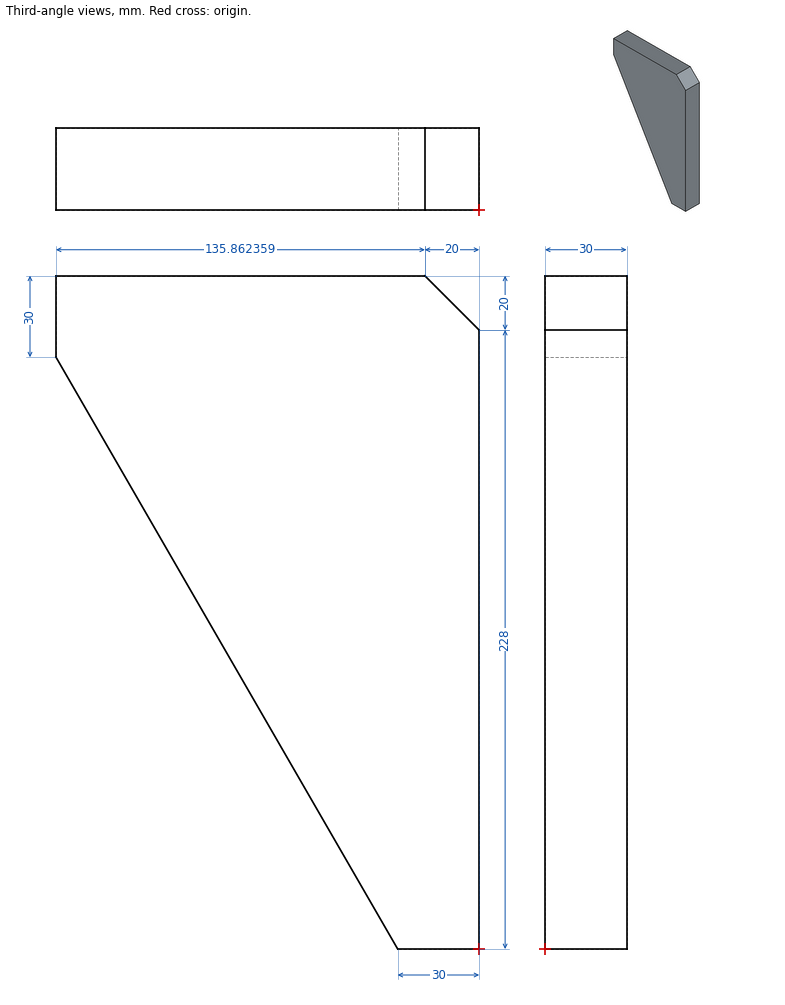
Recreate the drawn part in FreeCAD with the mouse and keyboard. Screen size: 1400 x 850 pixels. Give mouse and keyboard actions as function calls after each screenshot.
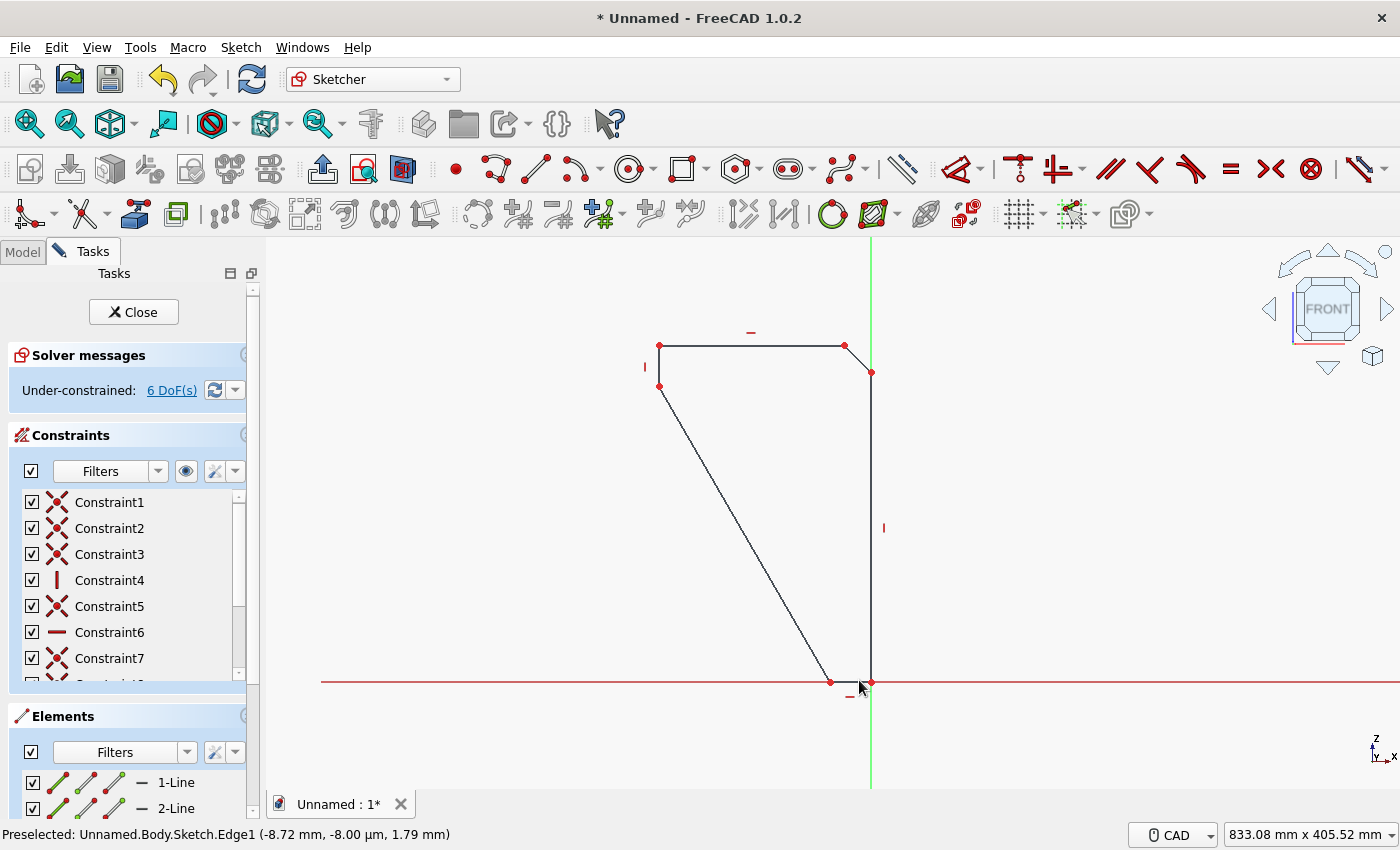
click(956, 170)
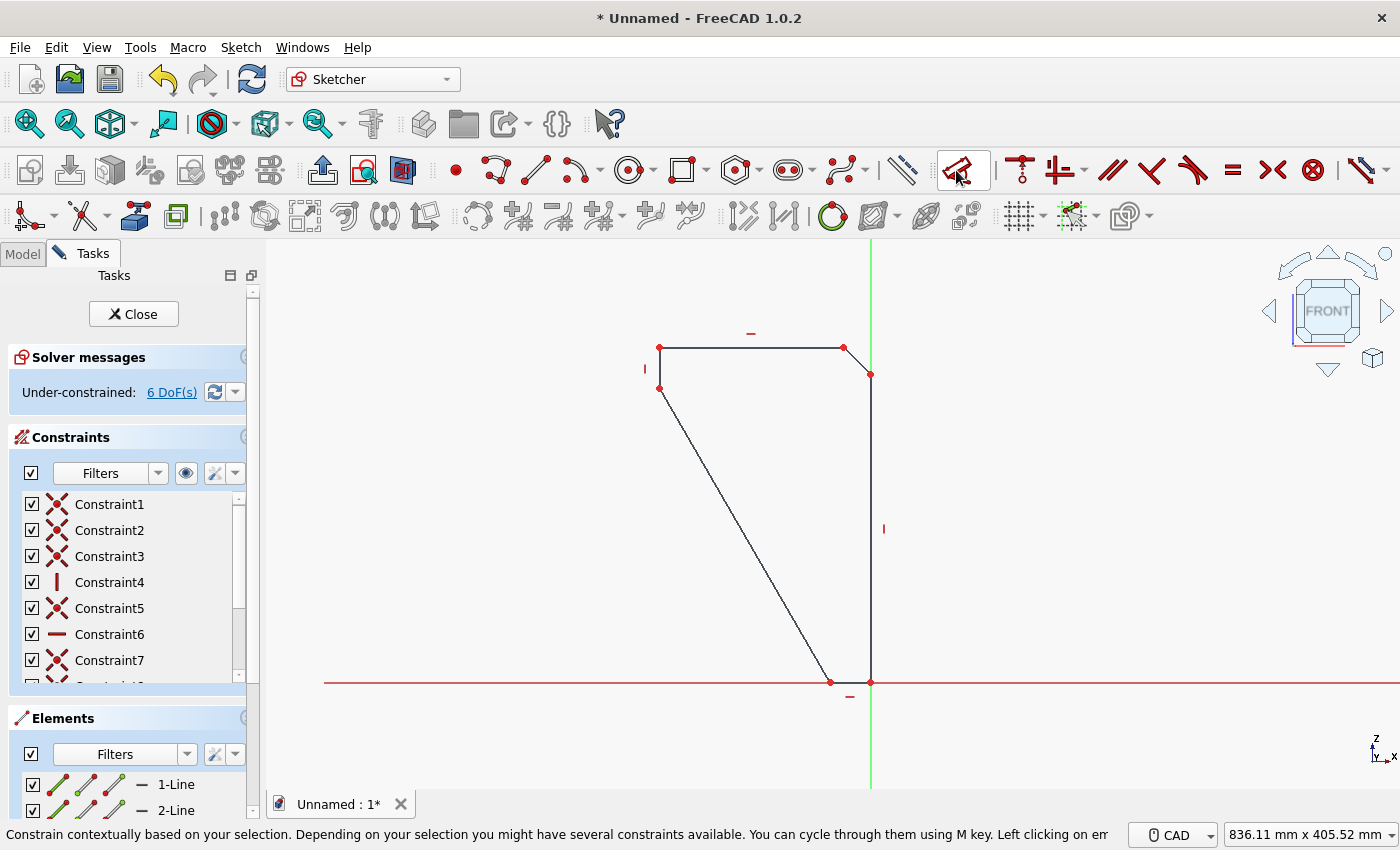
click(859, 683)
click(850, 717)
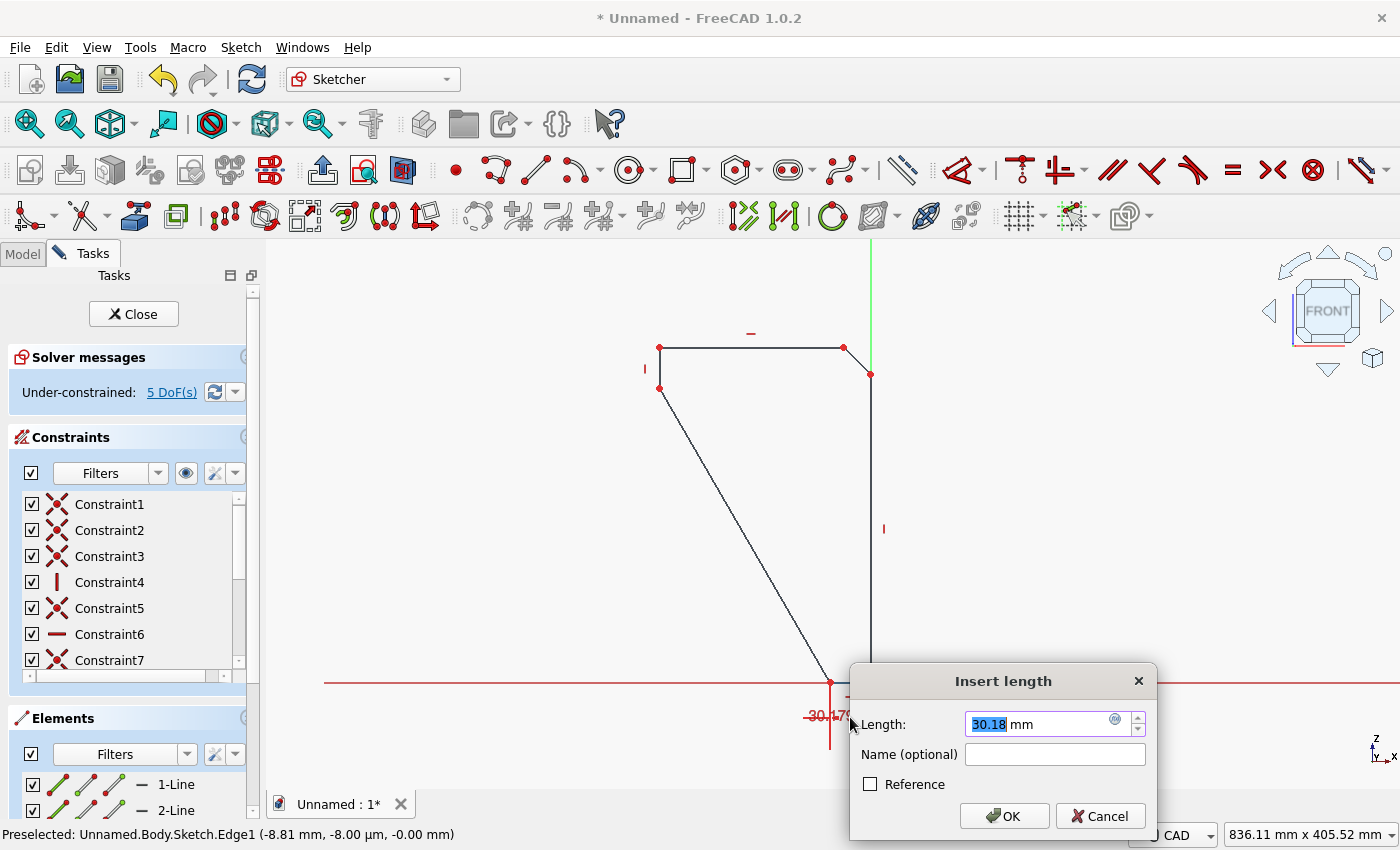
text(30)
key(Return)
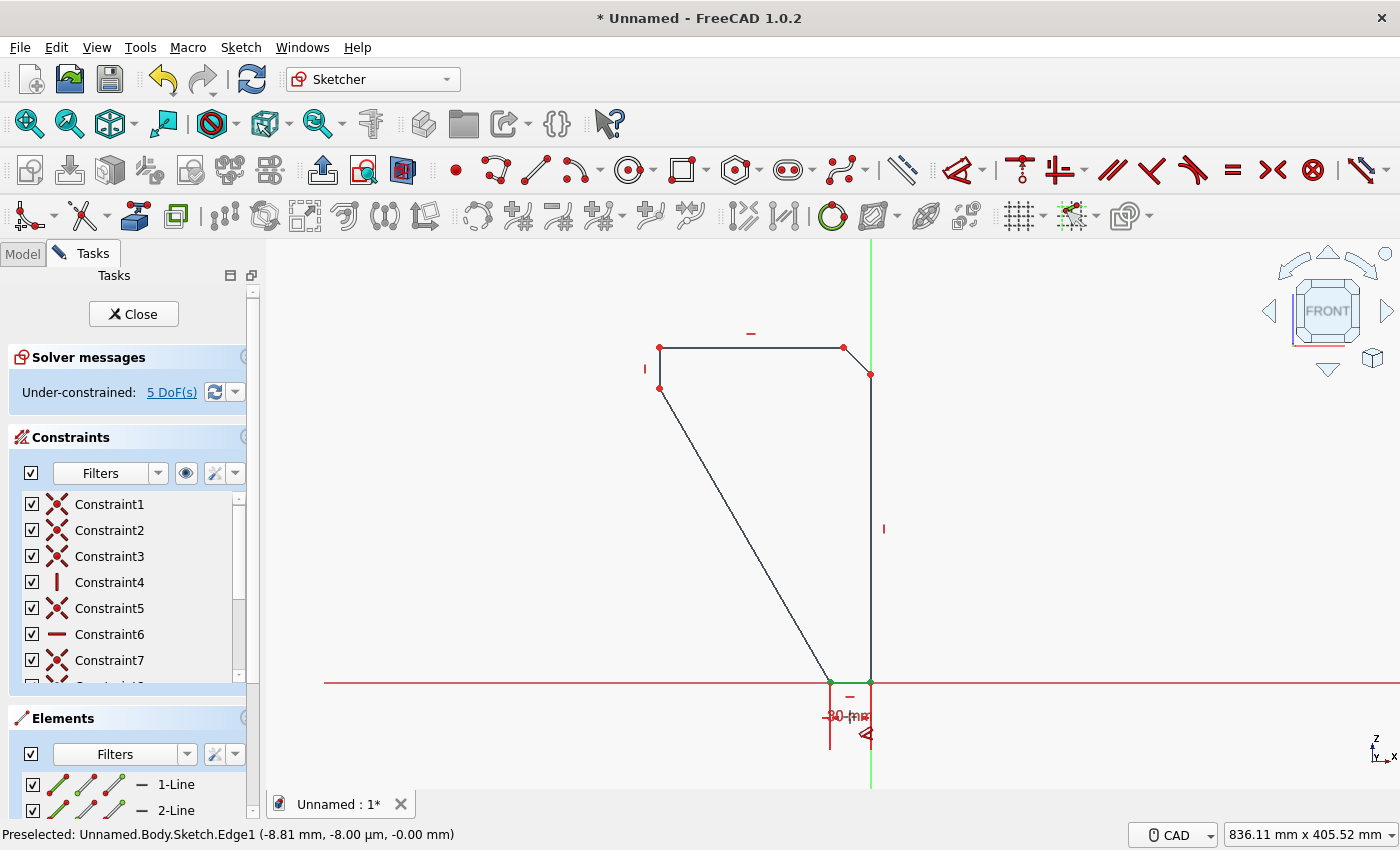
click(660, 376)
click(626, 368)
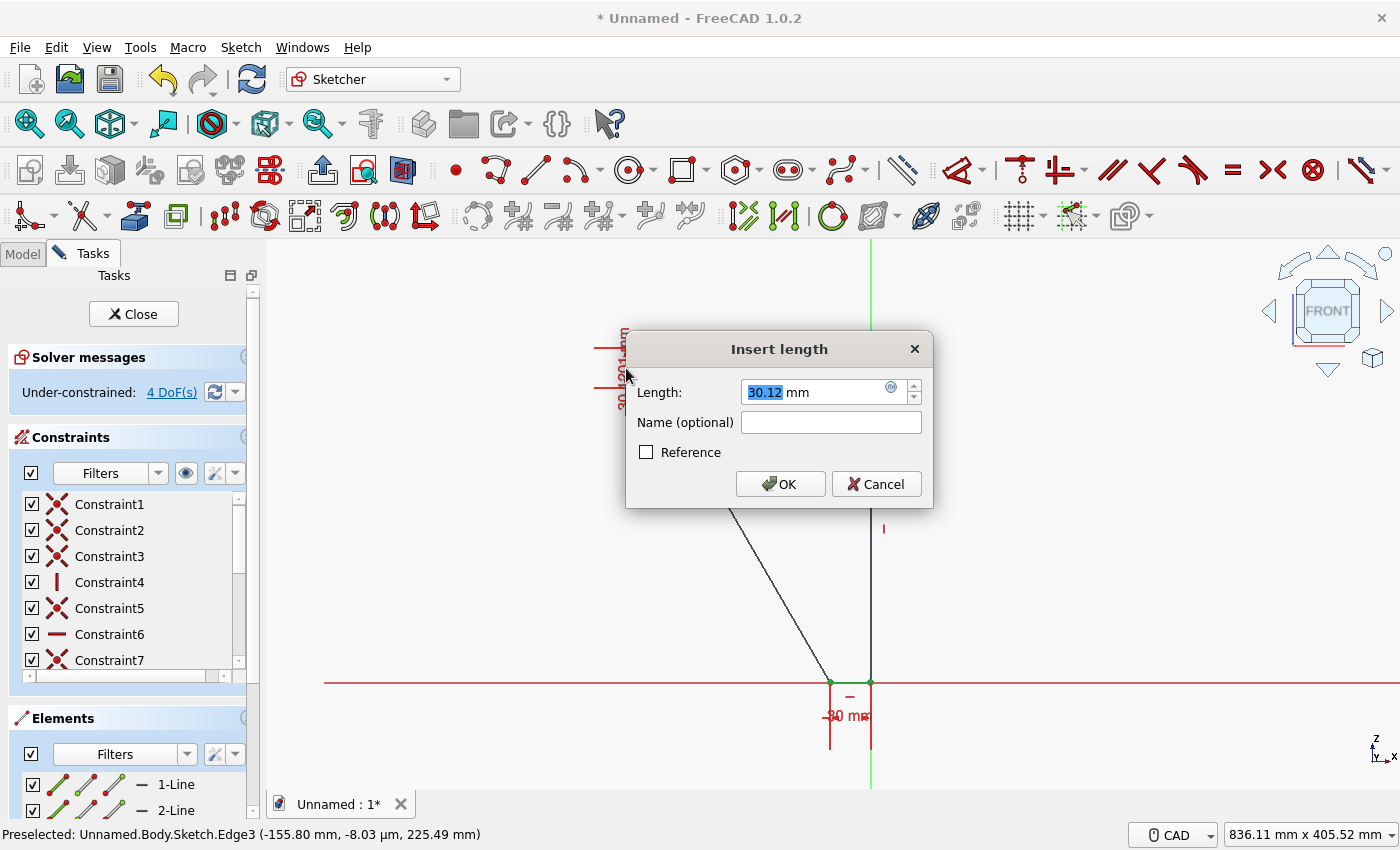
text(30)
key(Return)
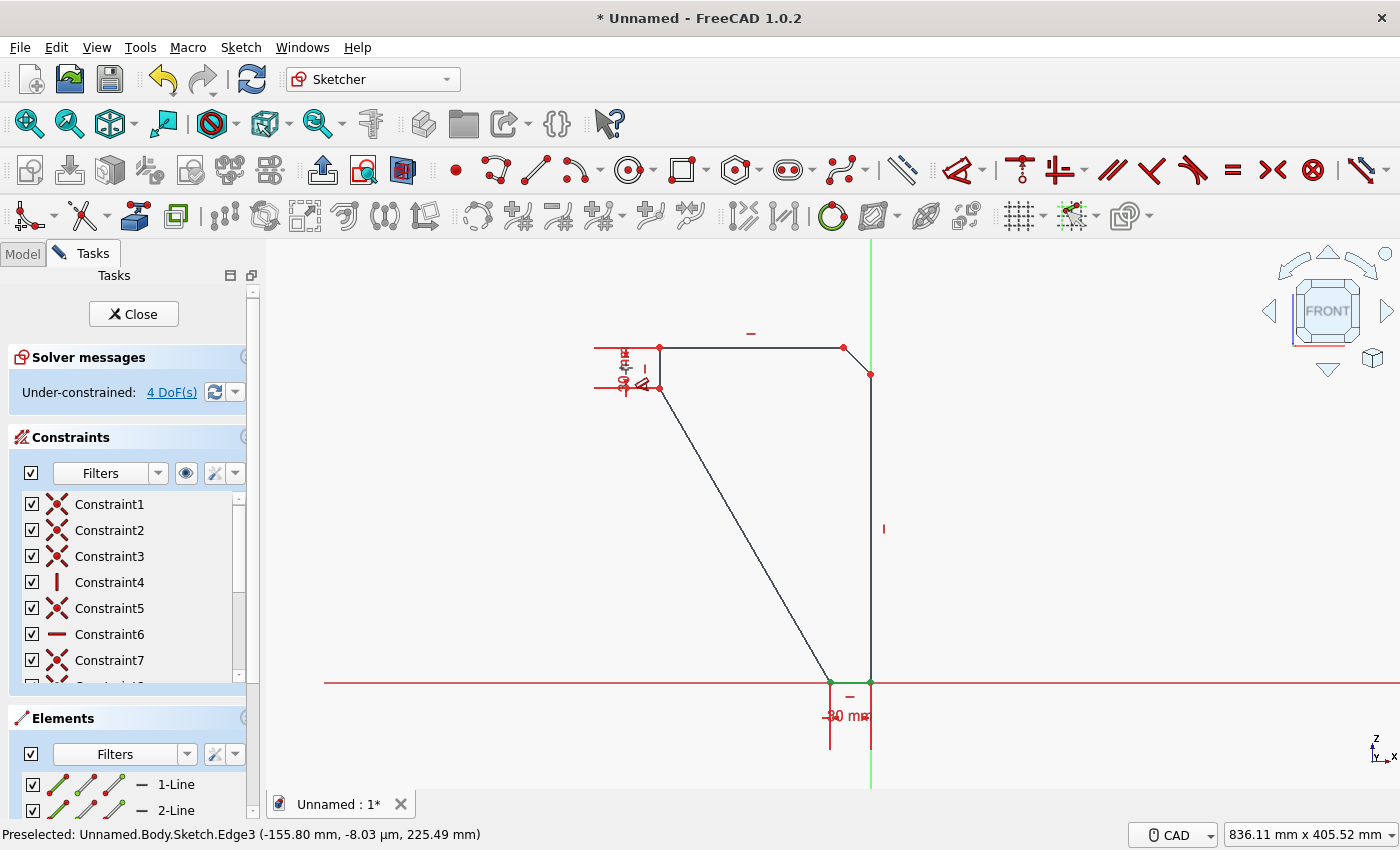
click(871, 467)
click(905, 529)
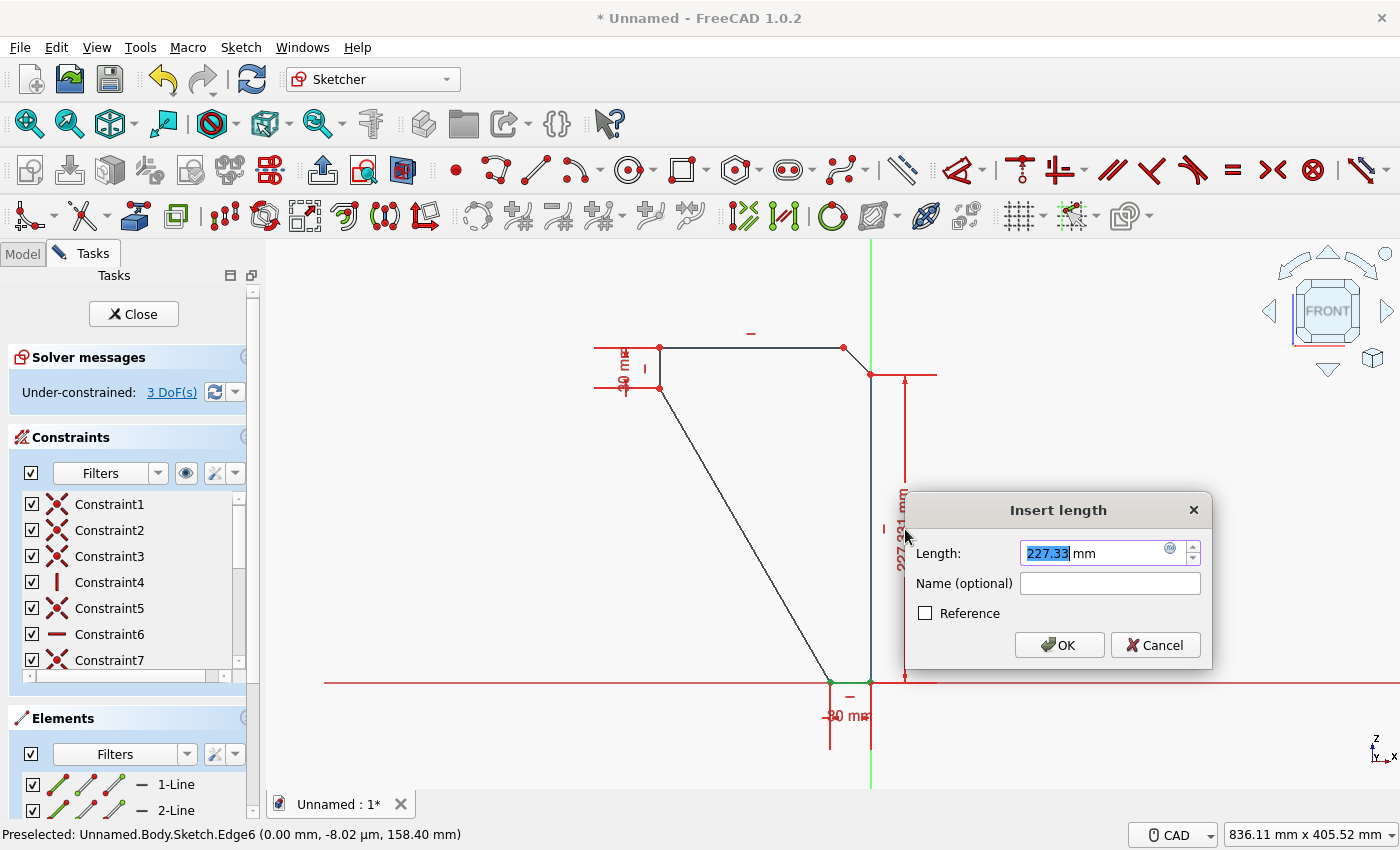
text(228)
key(Return)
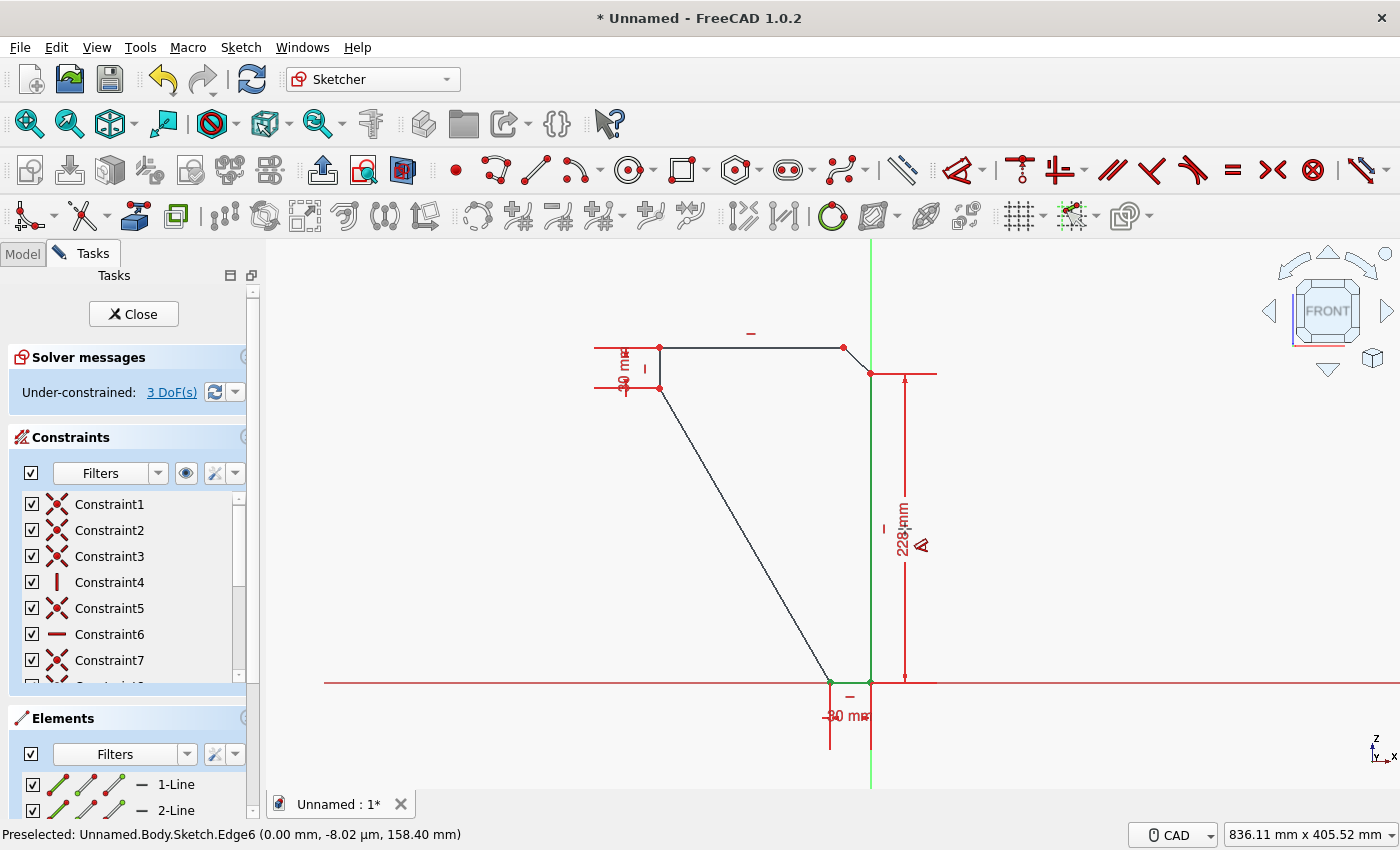
scroll(844, 348, up, 2)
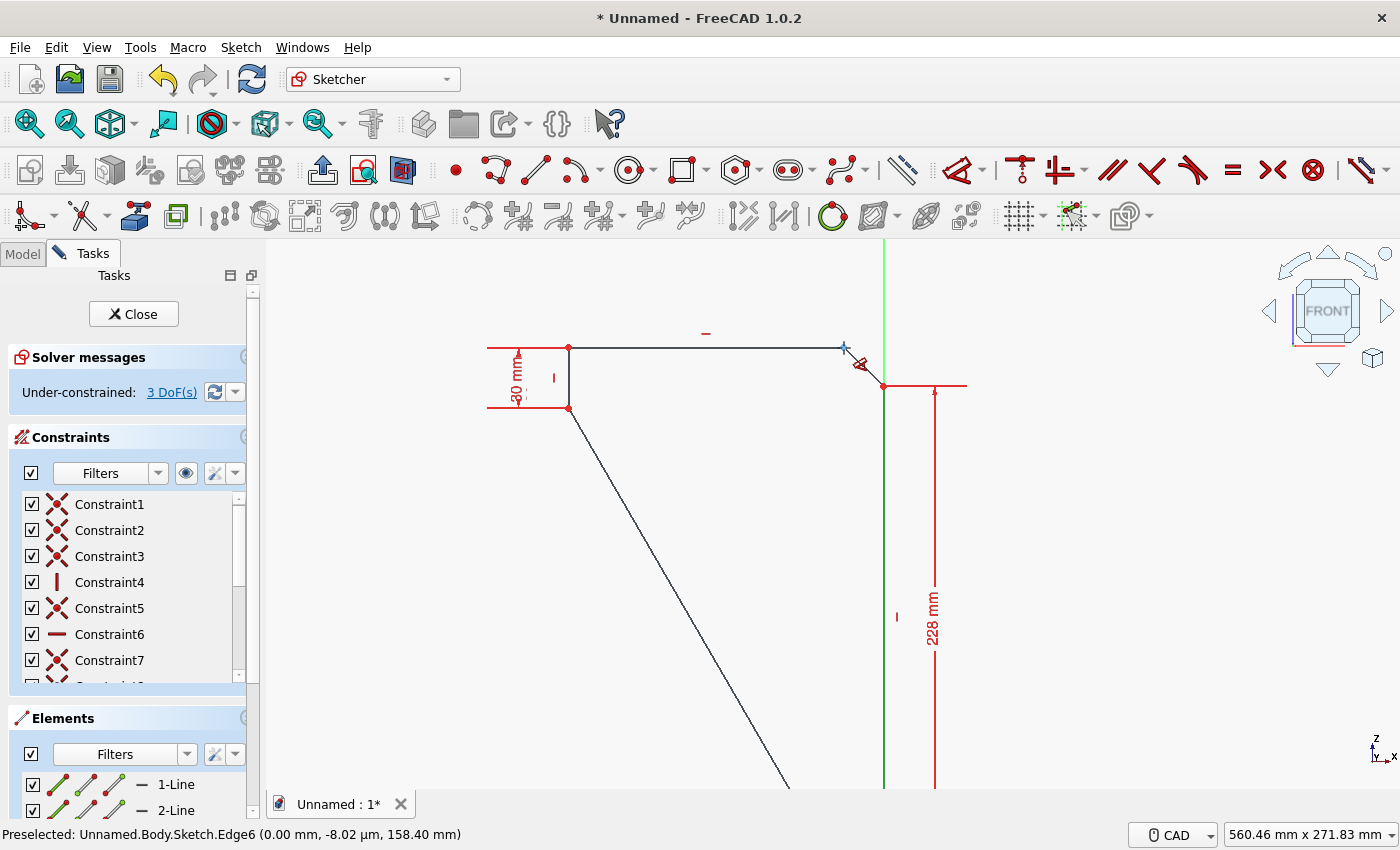
click(844, 348)
click(864, 314)